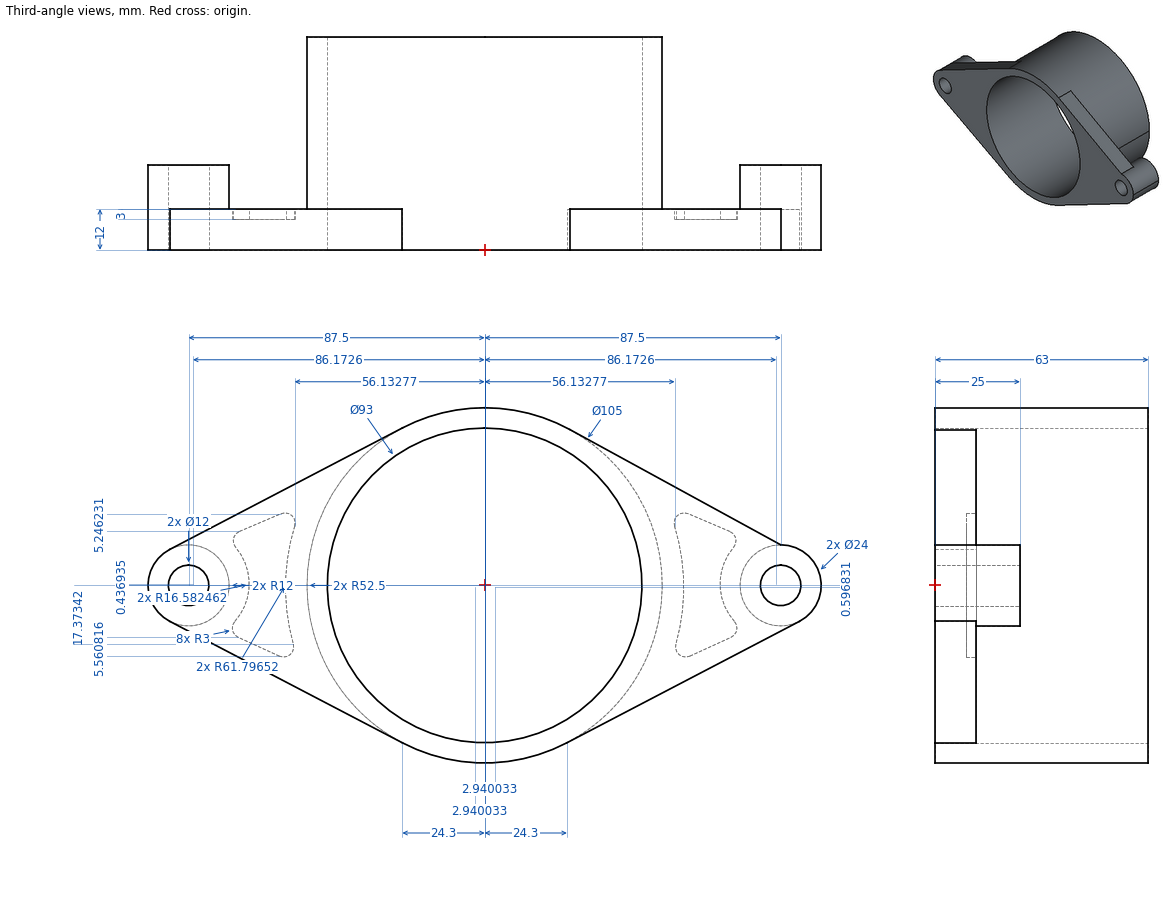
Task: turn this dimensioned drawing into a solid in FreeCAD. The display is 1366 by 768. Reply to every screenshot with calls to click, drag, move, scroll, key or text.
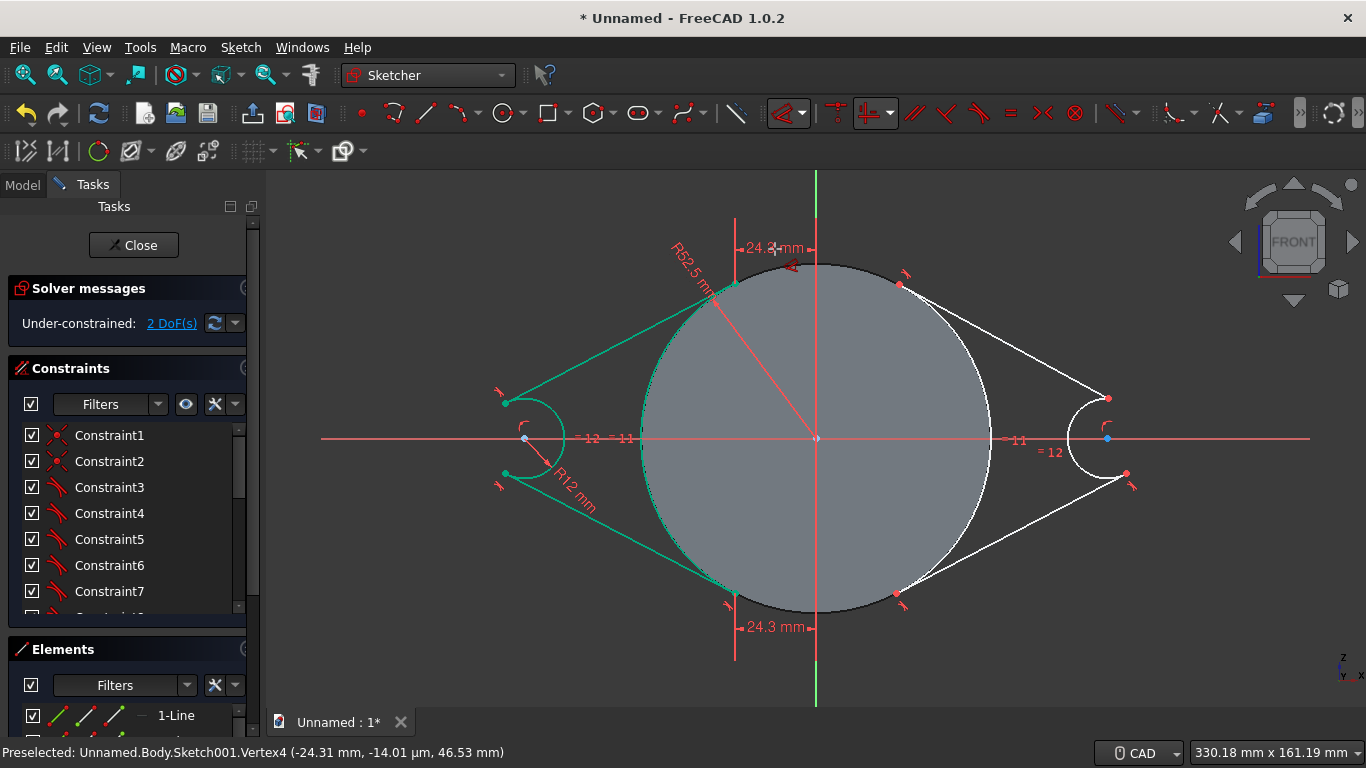
click(897, 594)
click(856, 628)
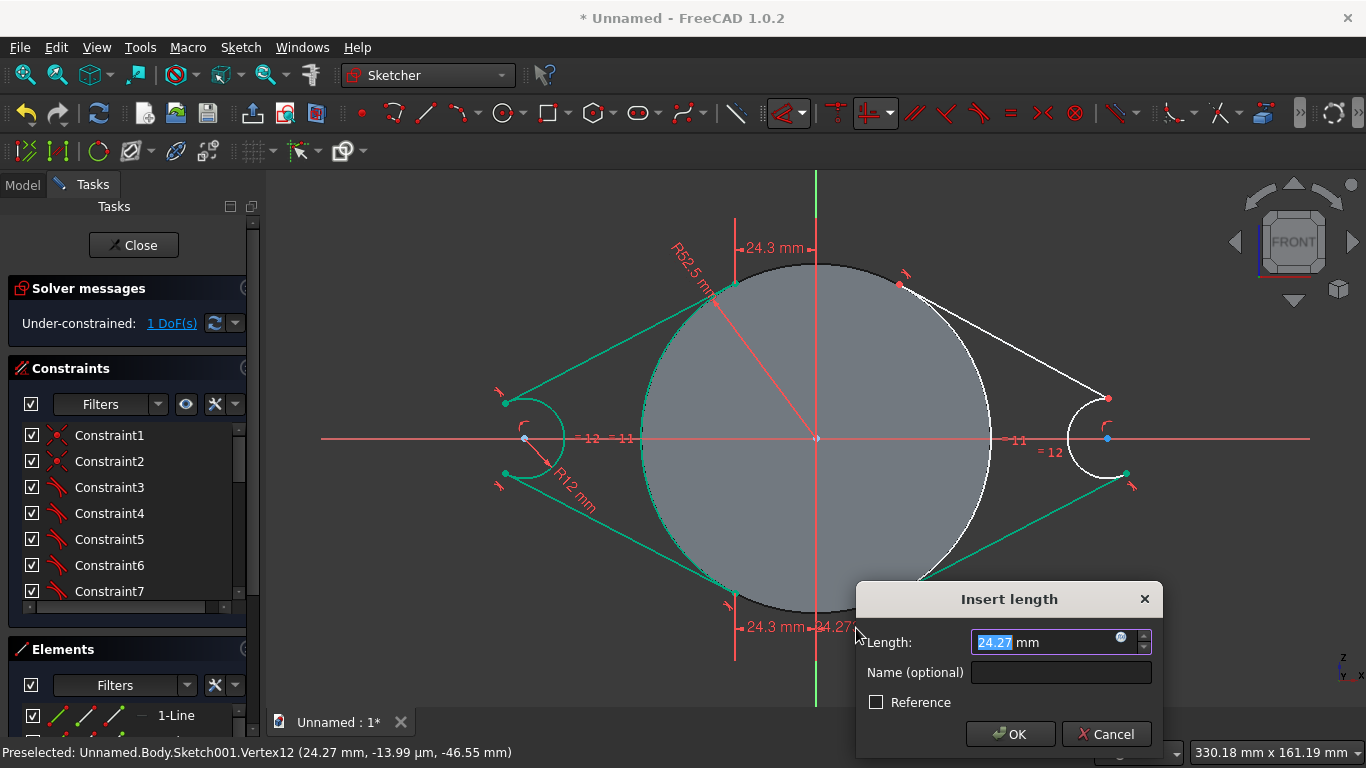
text(24.3)
key(Return)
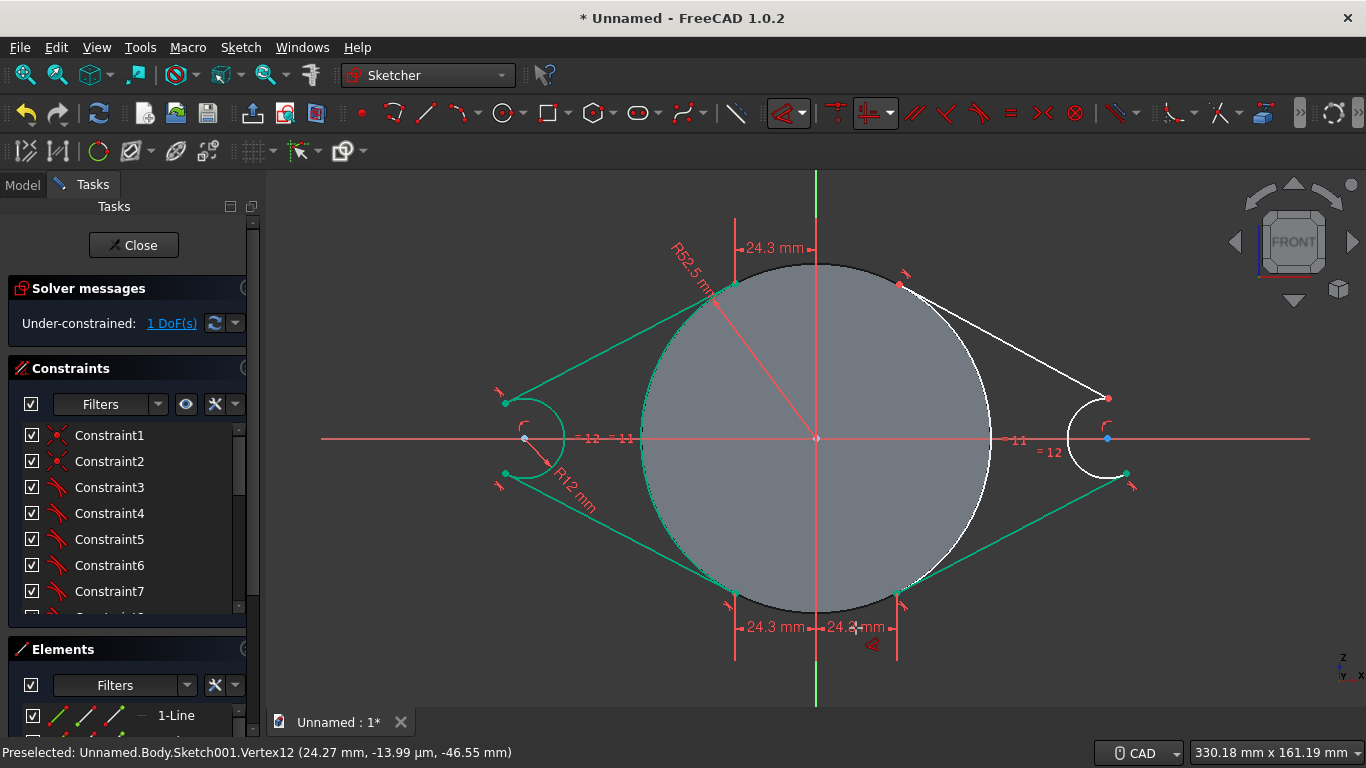
click(1108, 399)
click(895, 365)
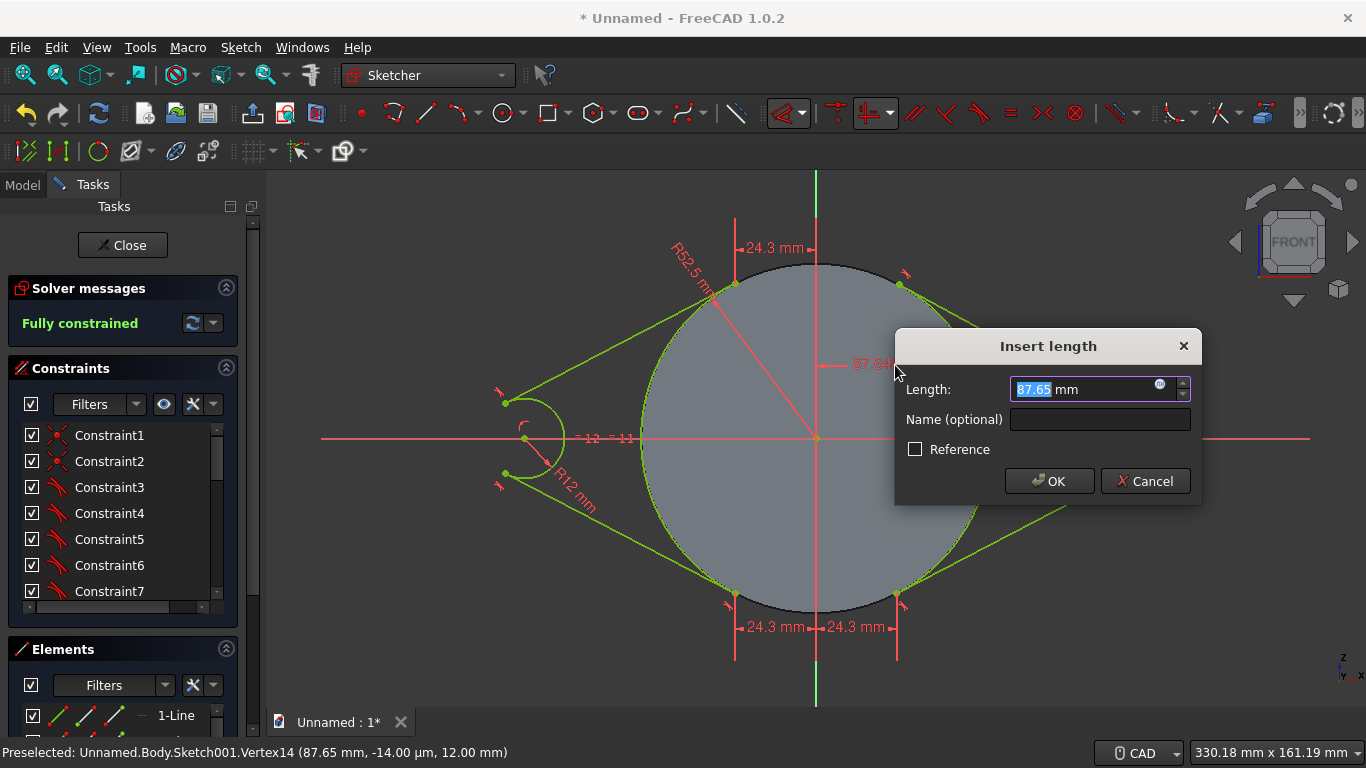
text(87.5)
key(Return)
key(Escape)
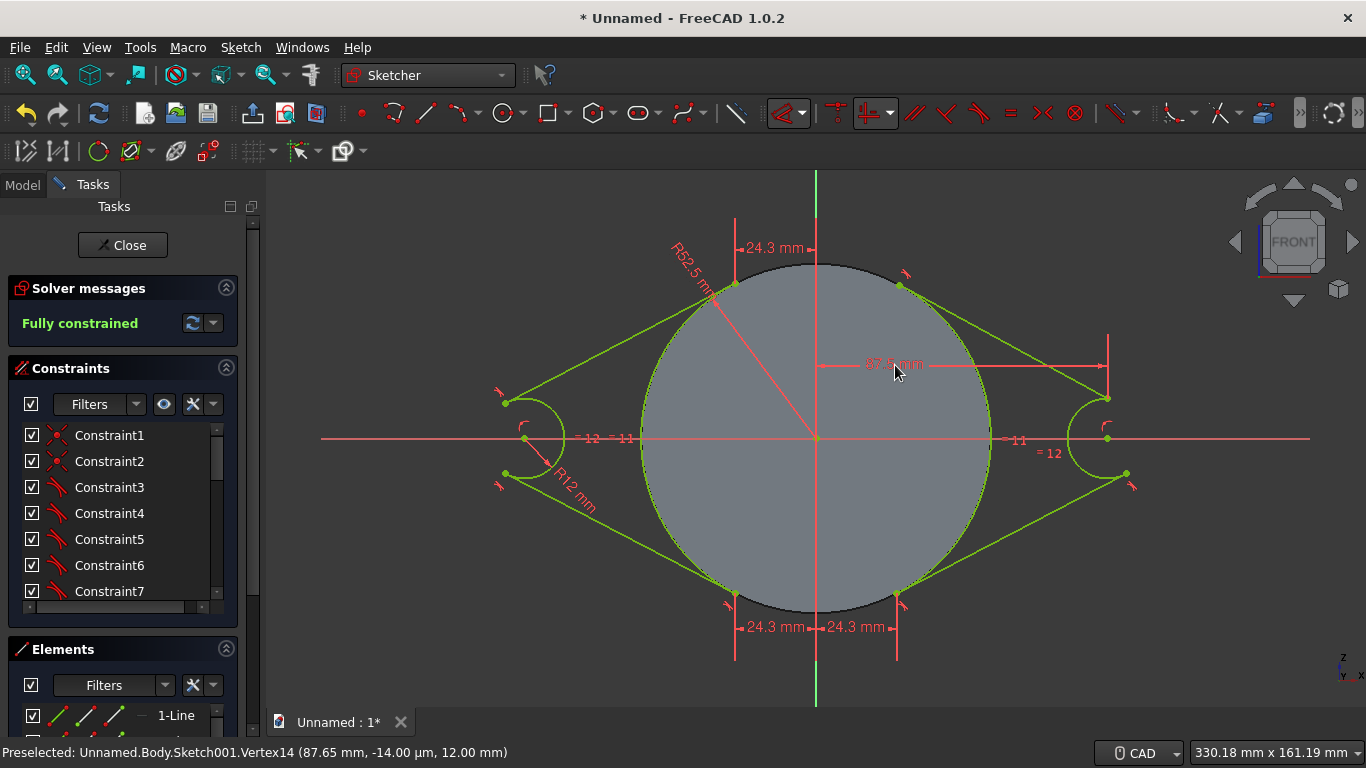
click(123, 245)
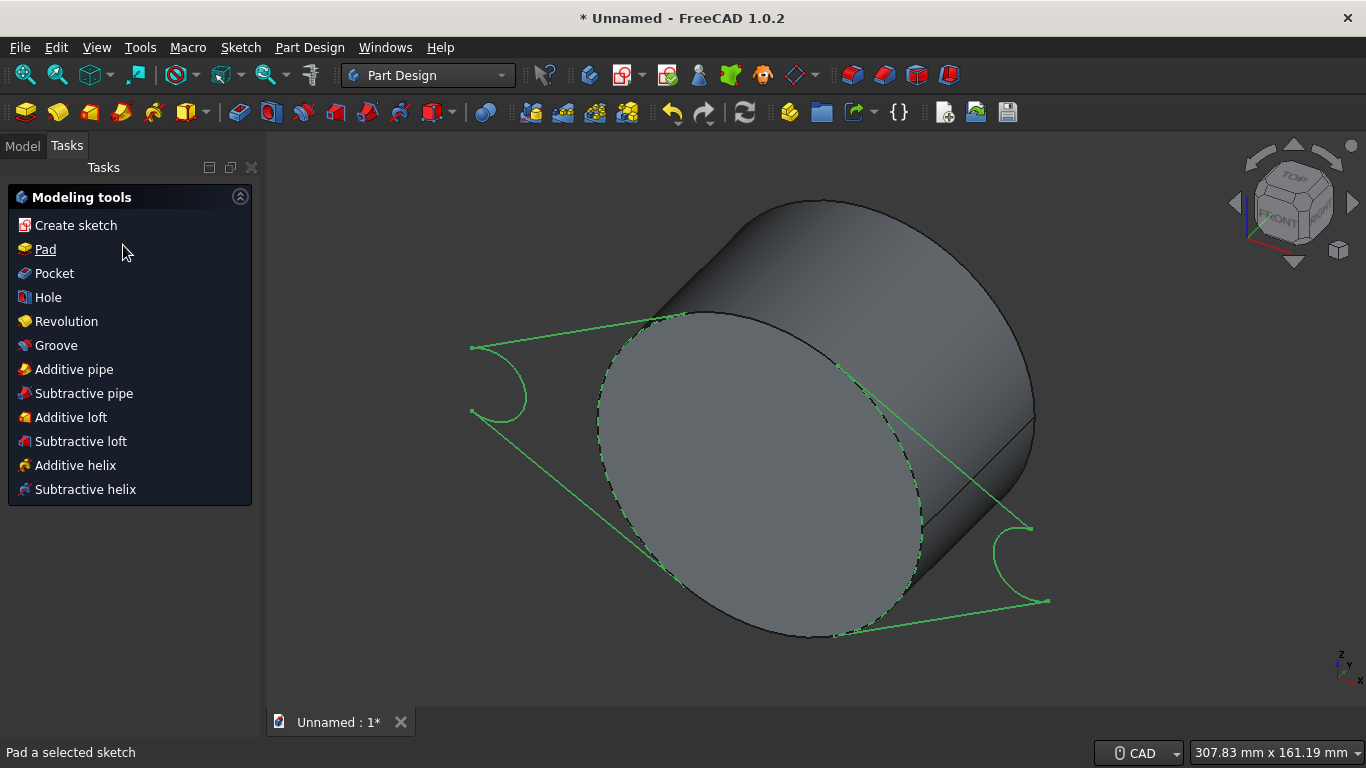
click(26, 112)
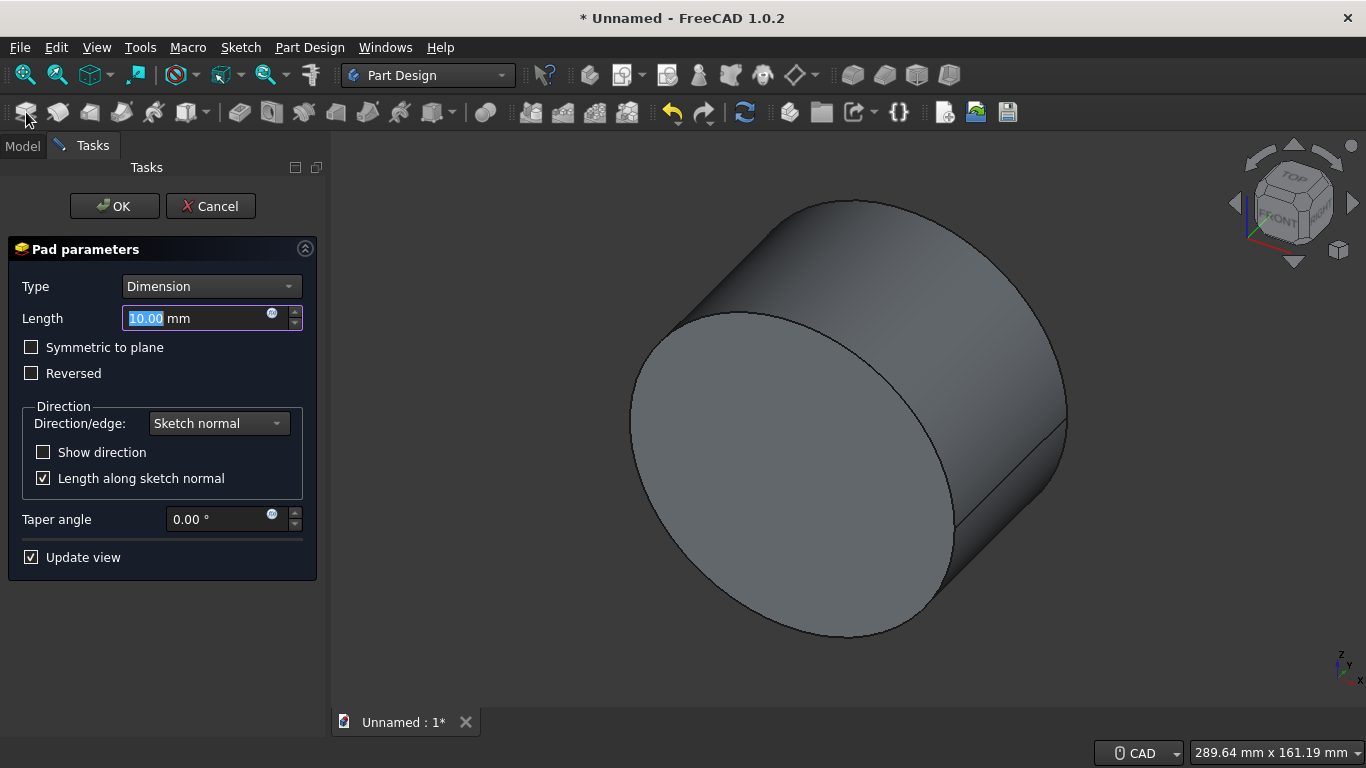
text(12)
key(Tab)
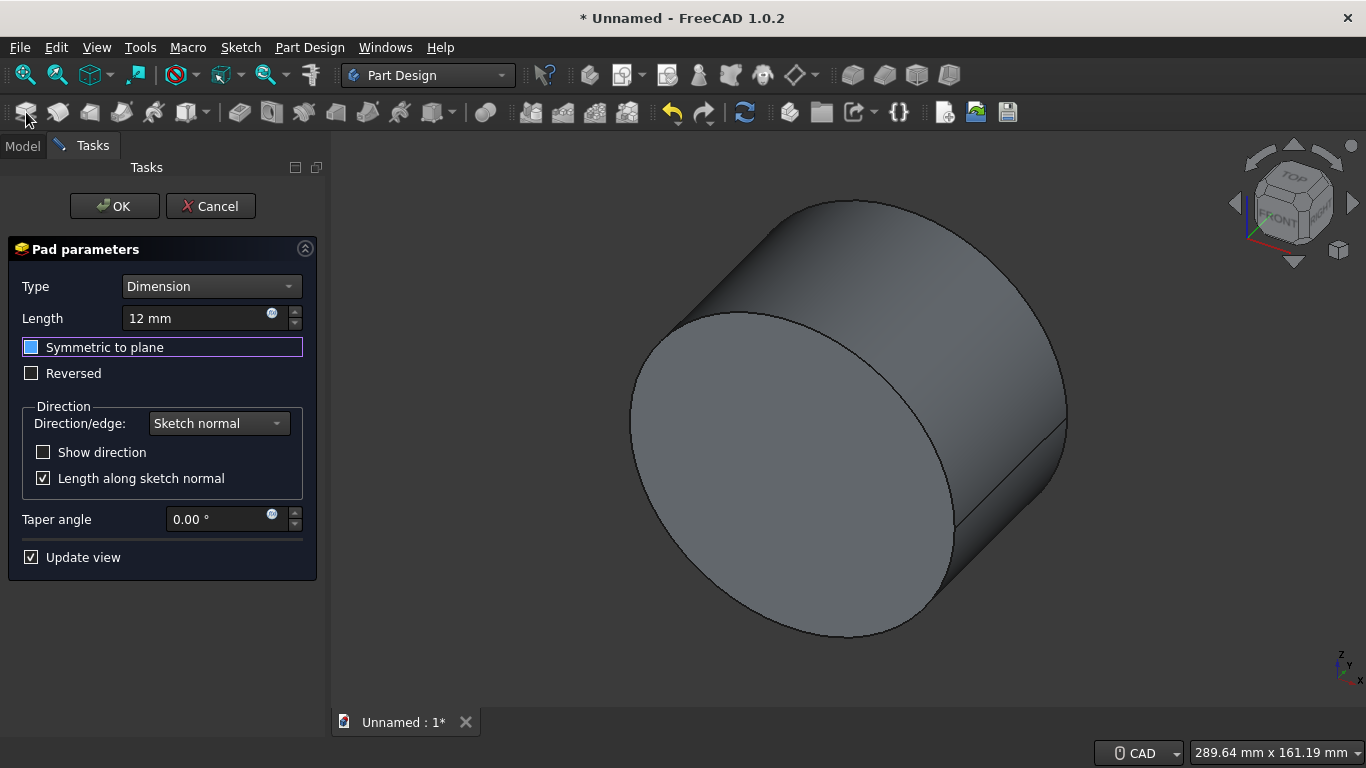
click(30, 373)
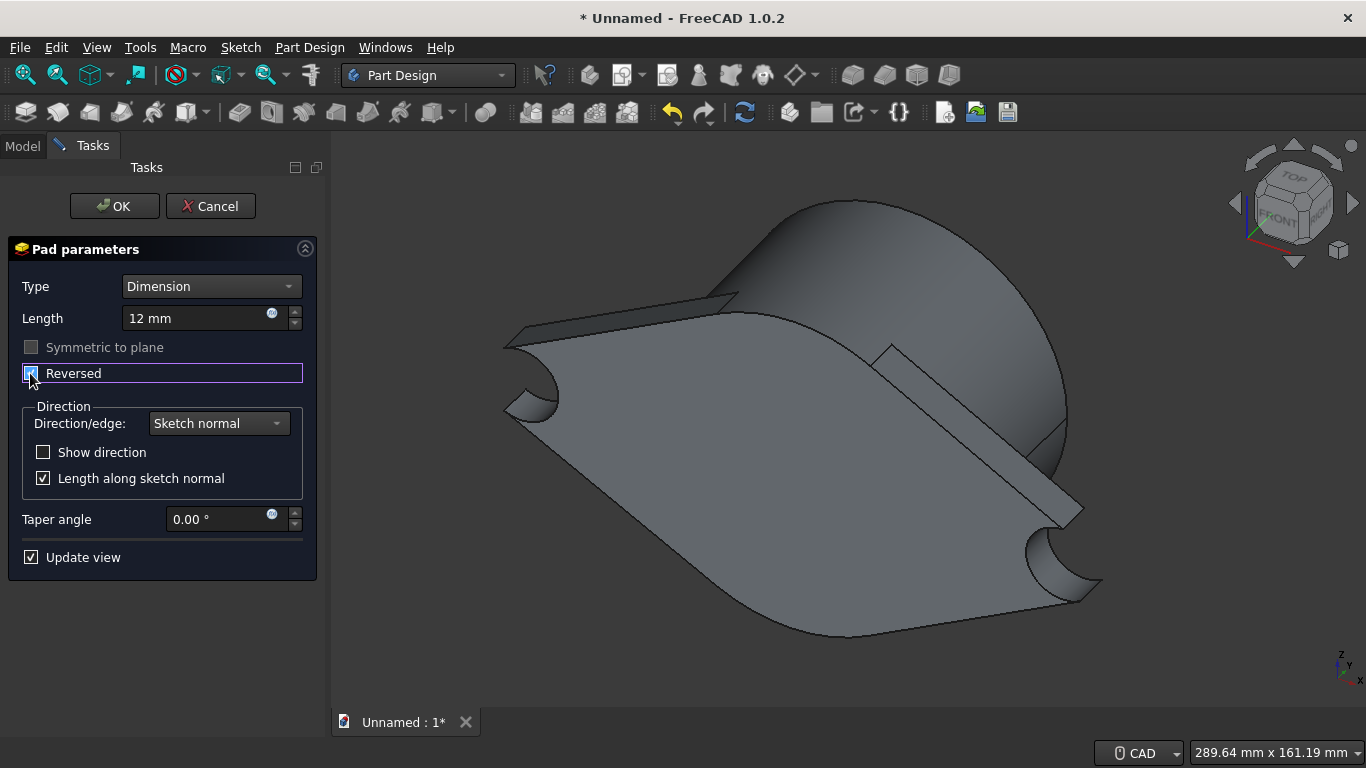
click(115, 206)